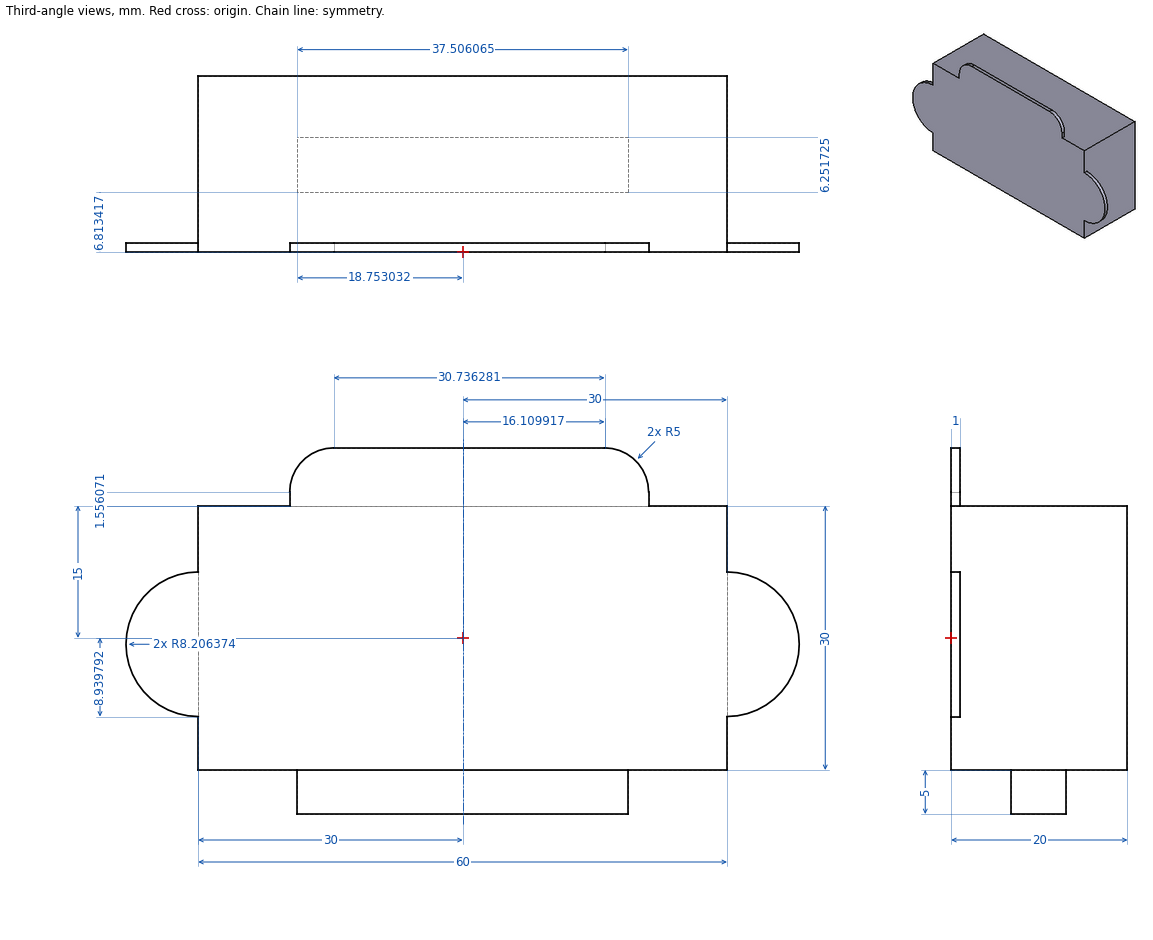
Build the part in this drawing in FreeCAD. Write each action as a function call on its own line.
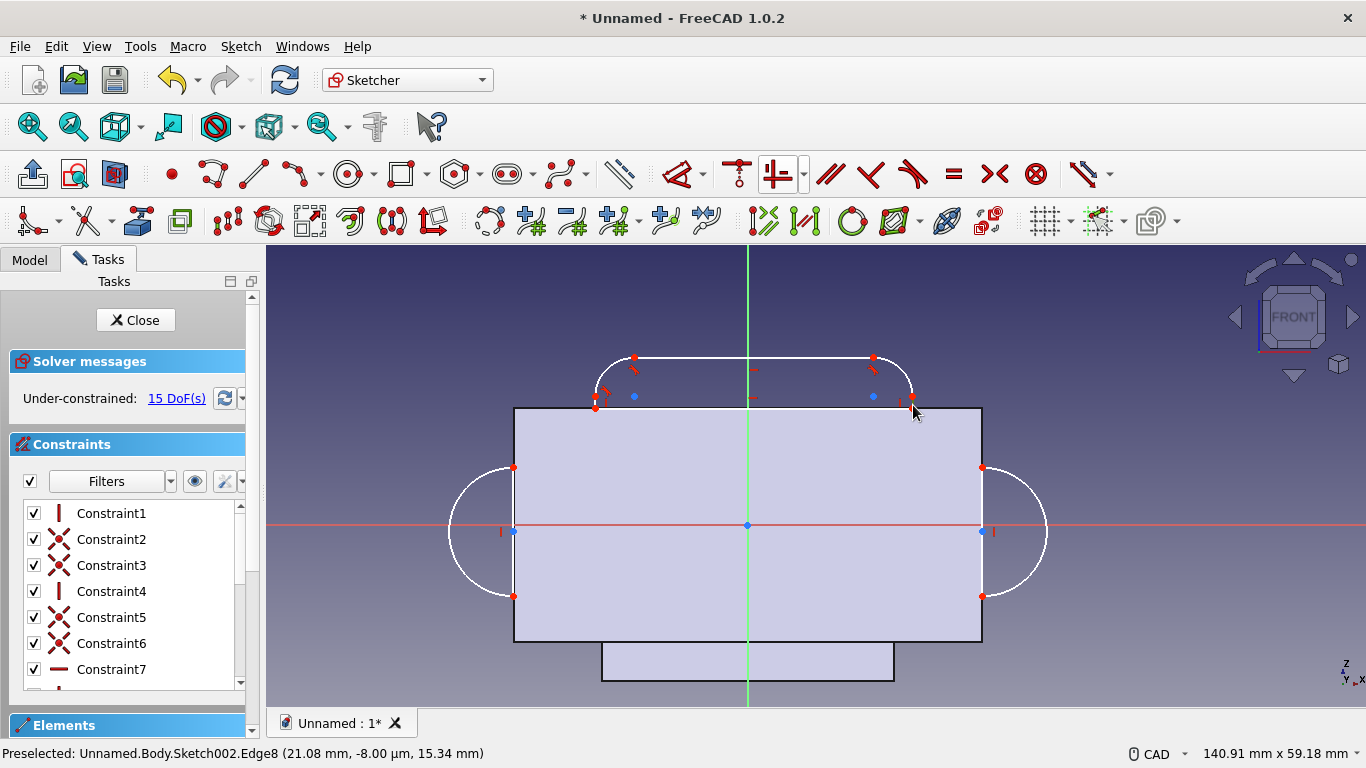
click(908, 379)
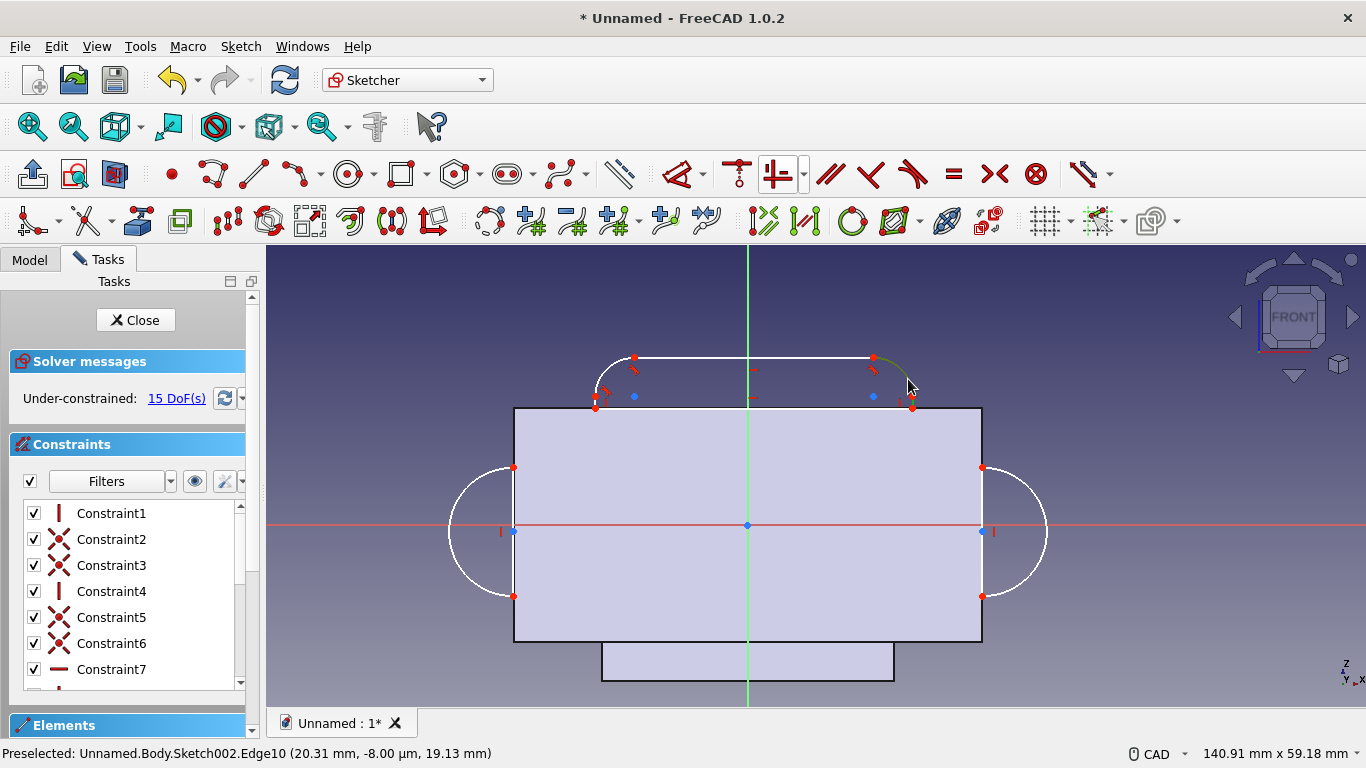
click(913, 174)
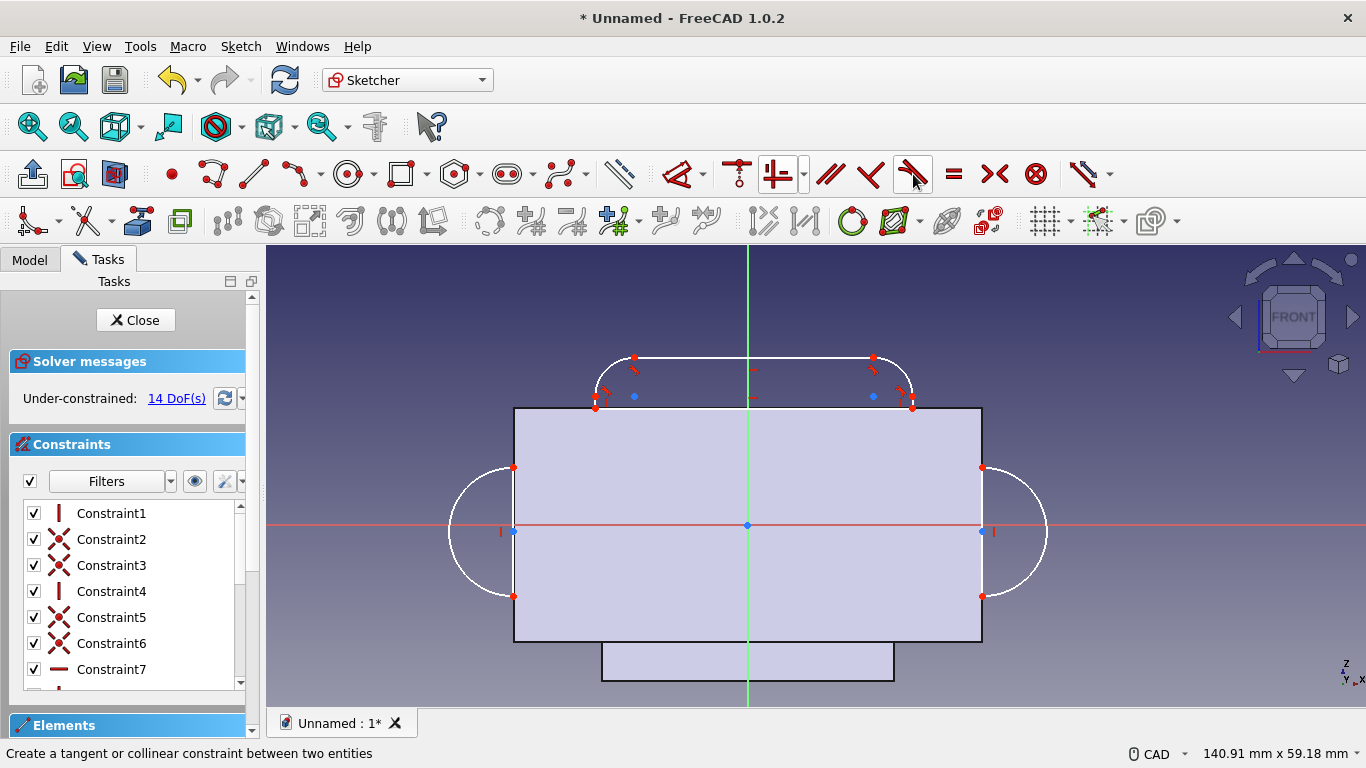
click(461, 494)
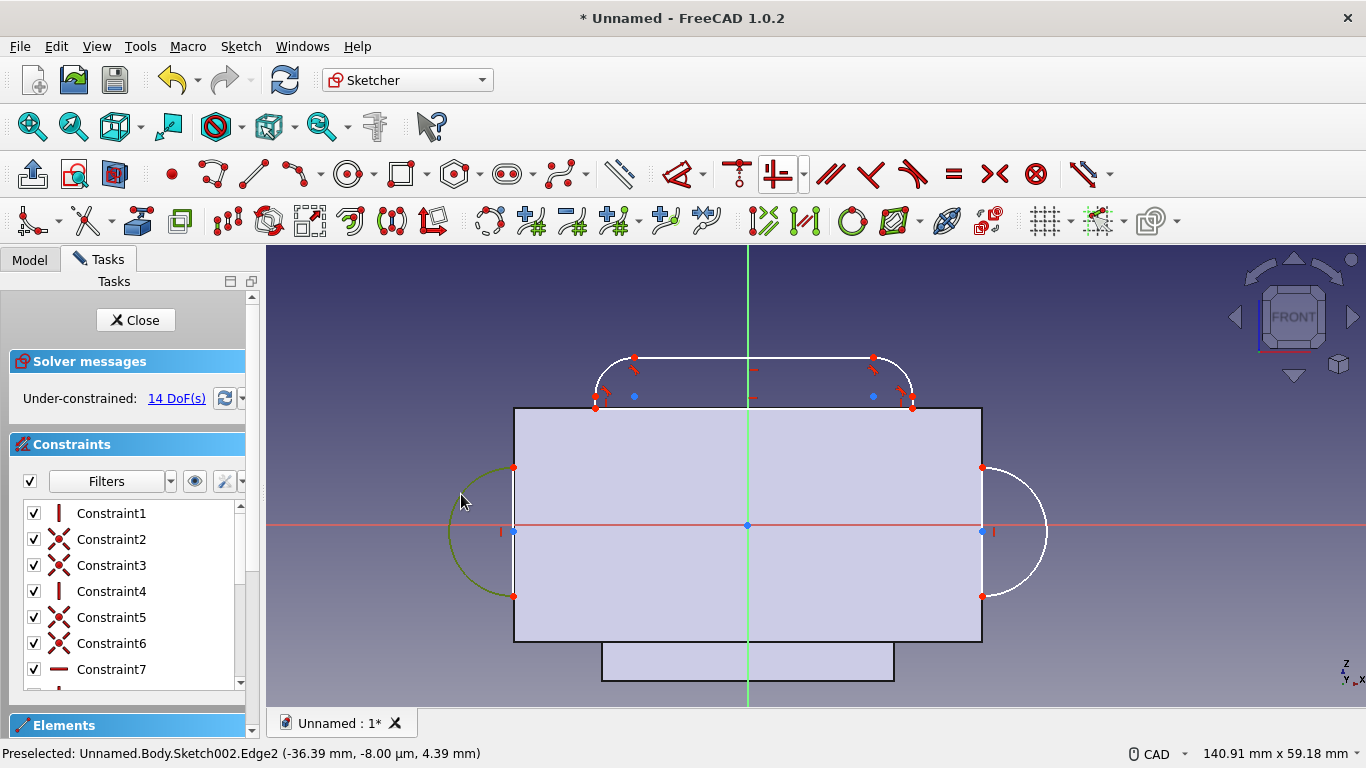
click(1034, 570)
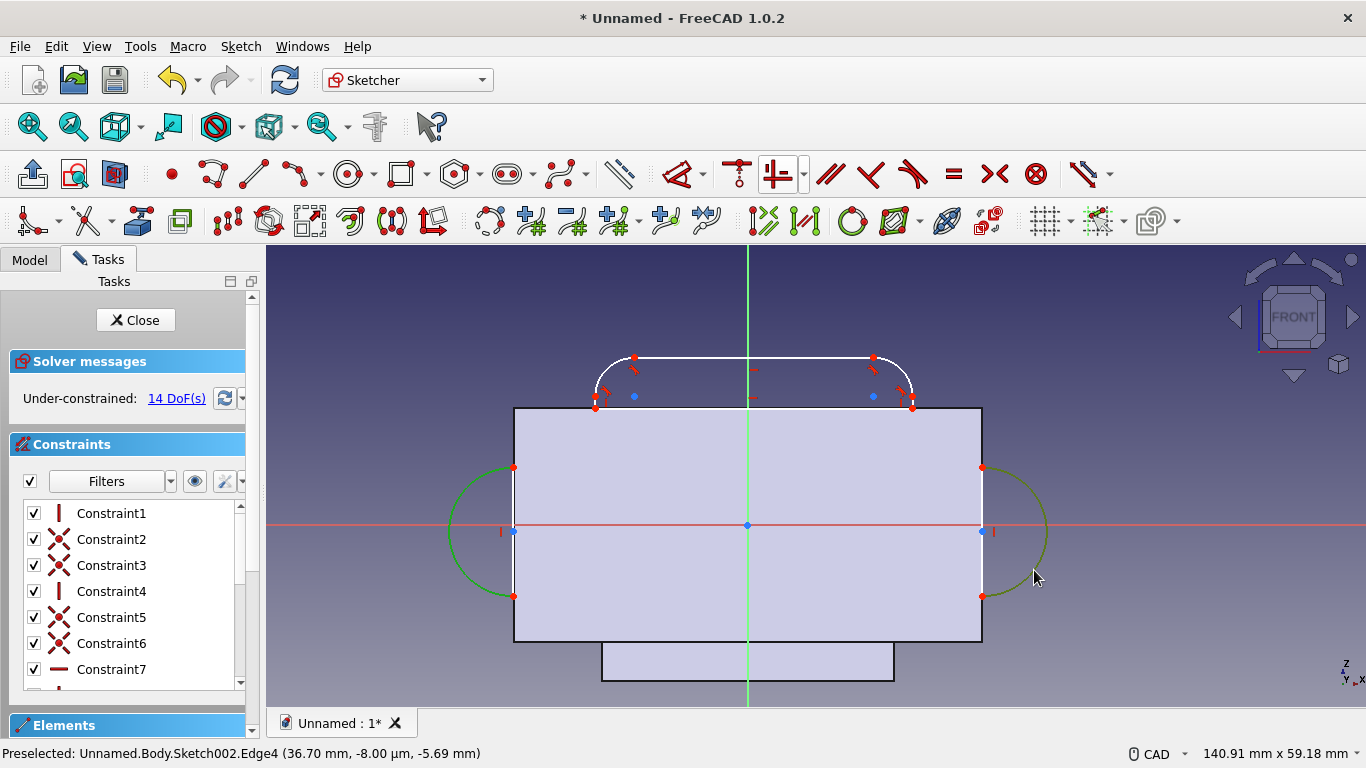
key(e)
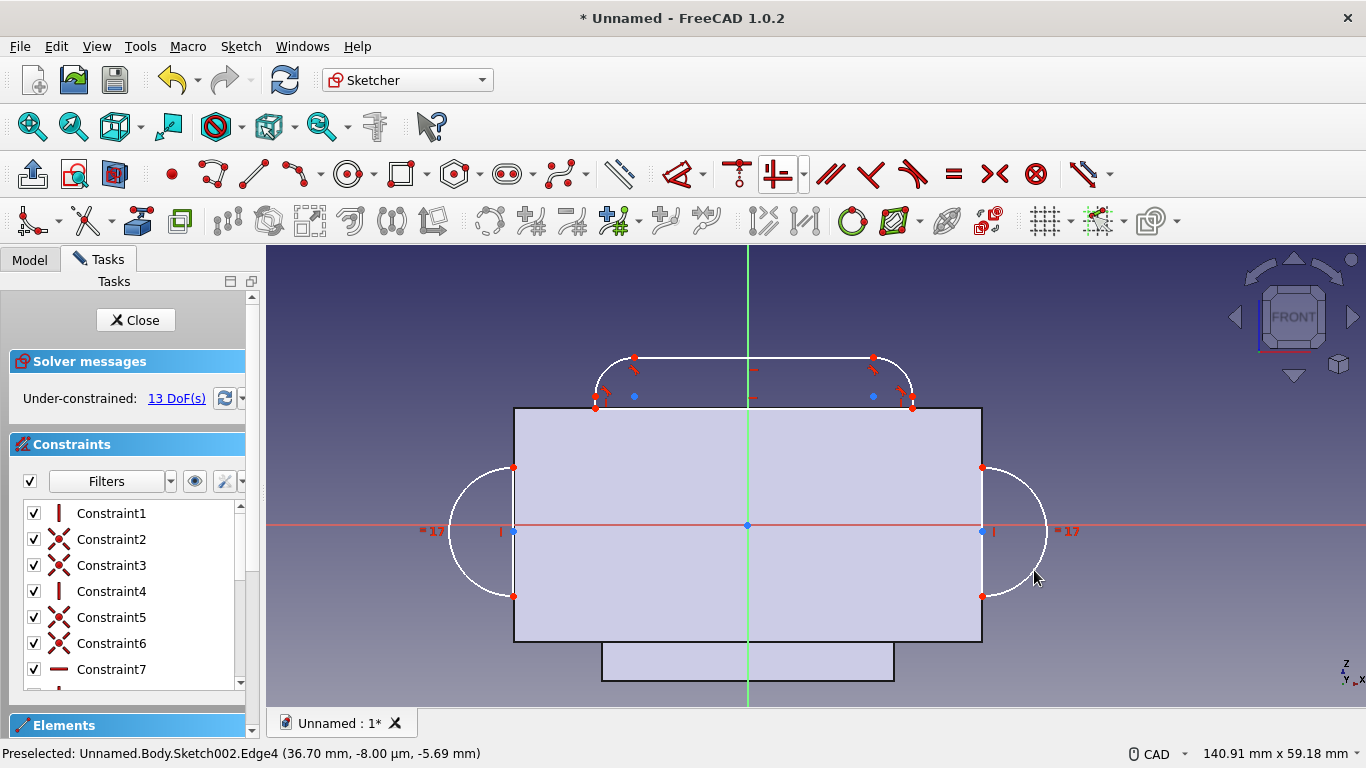
click(617, 362)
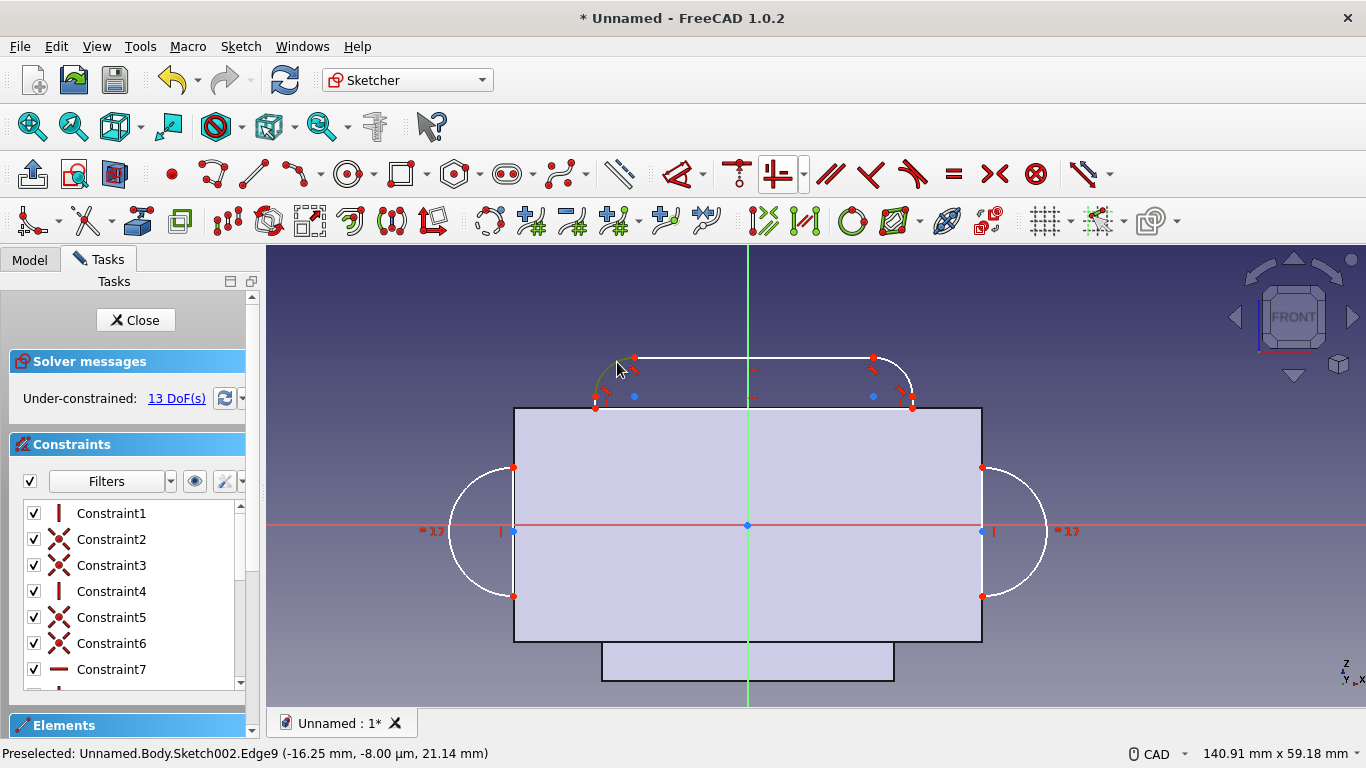
click(908, 379)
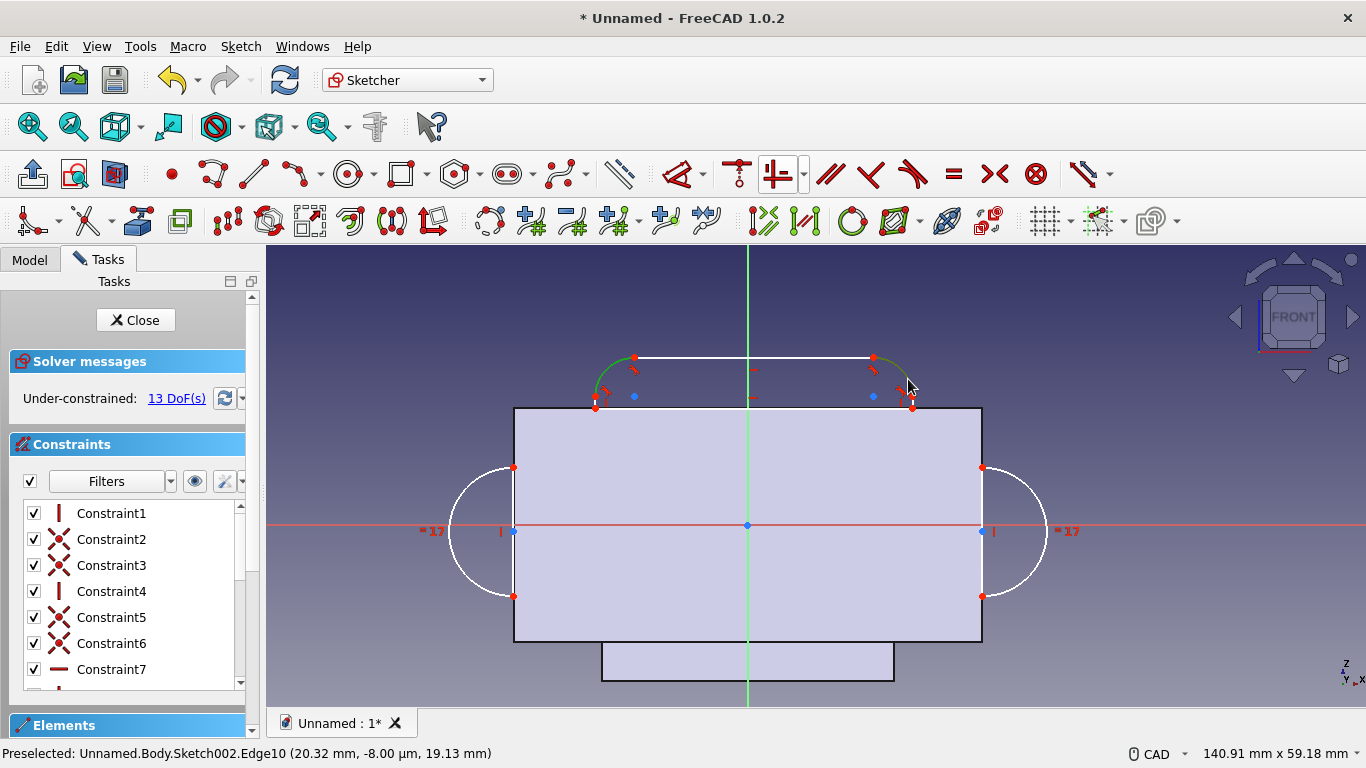
key(e)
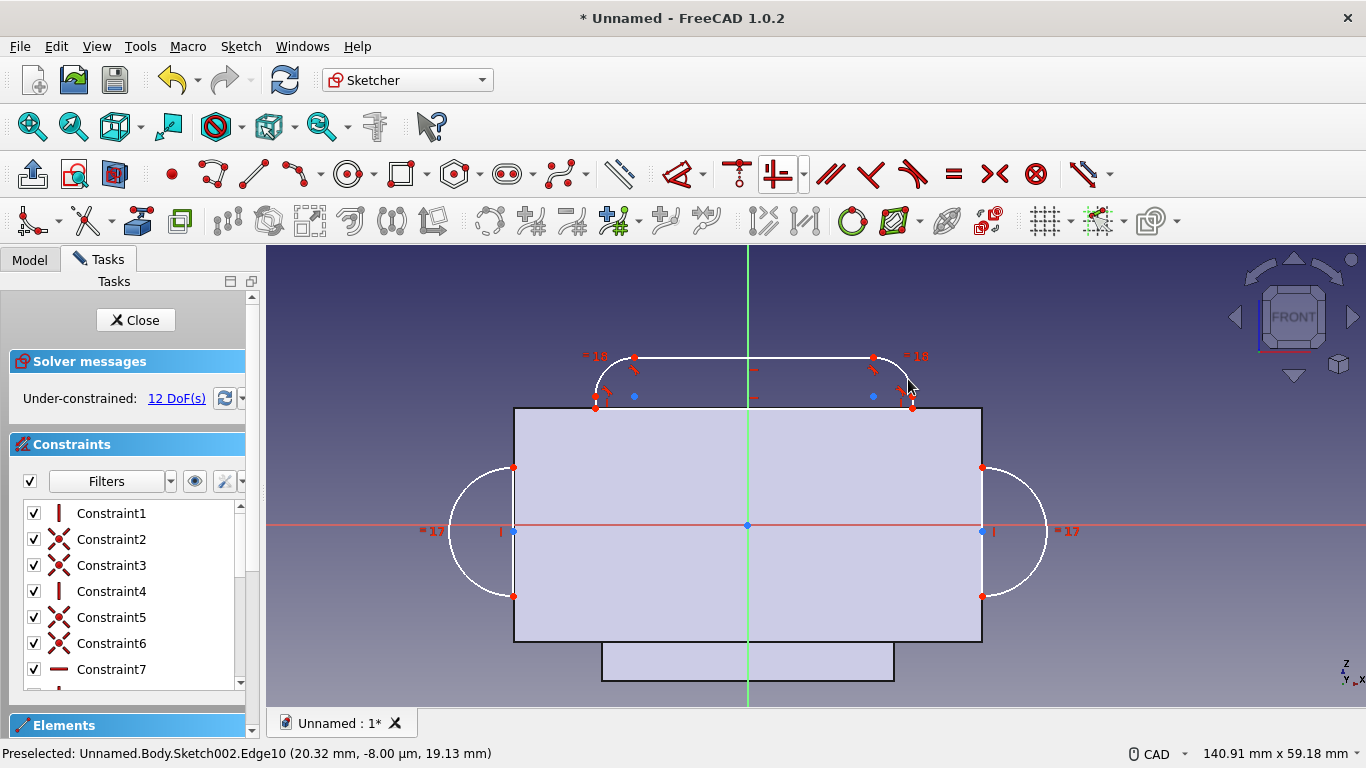
click(513, 532)